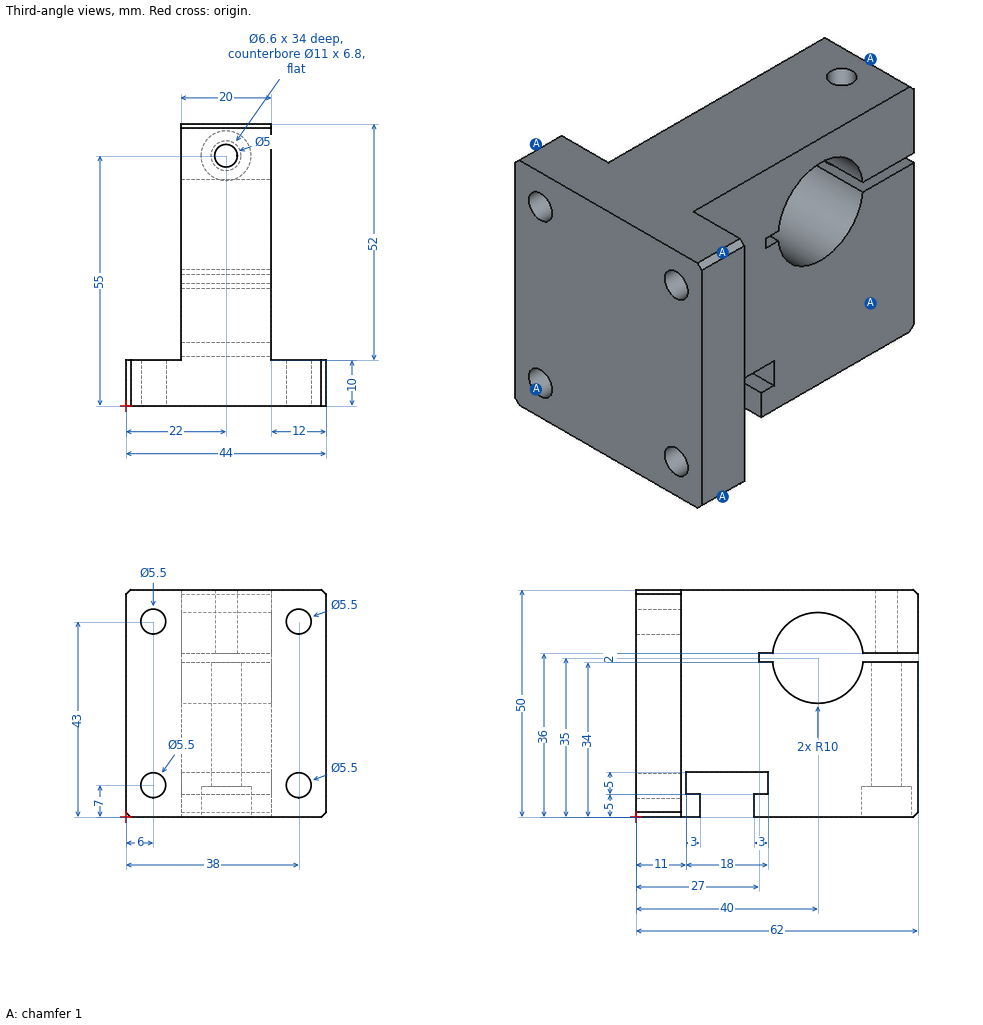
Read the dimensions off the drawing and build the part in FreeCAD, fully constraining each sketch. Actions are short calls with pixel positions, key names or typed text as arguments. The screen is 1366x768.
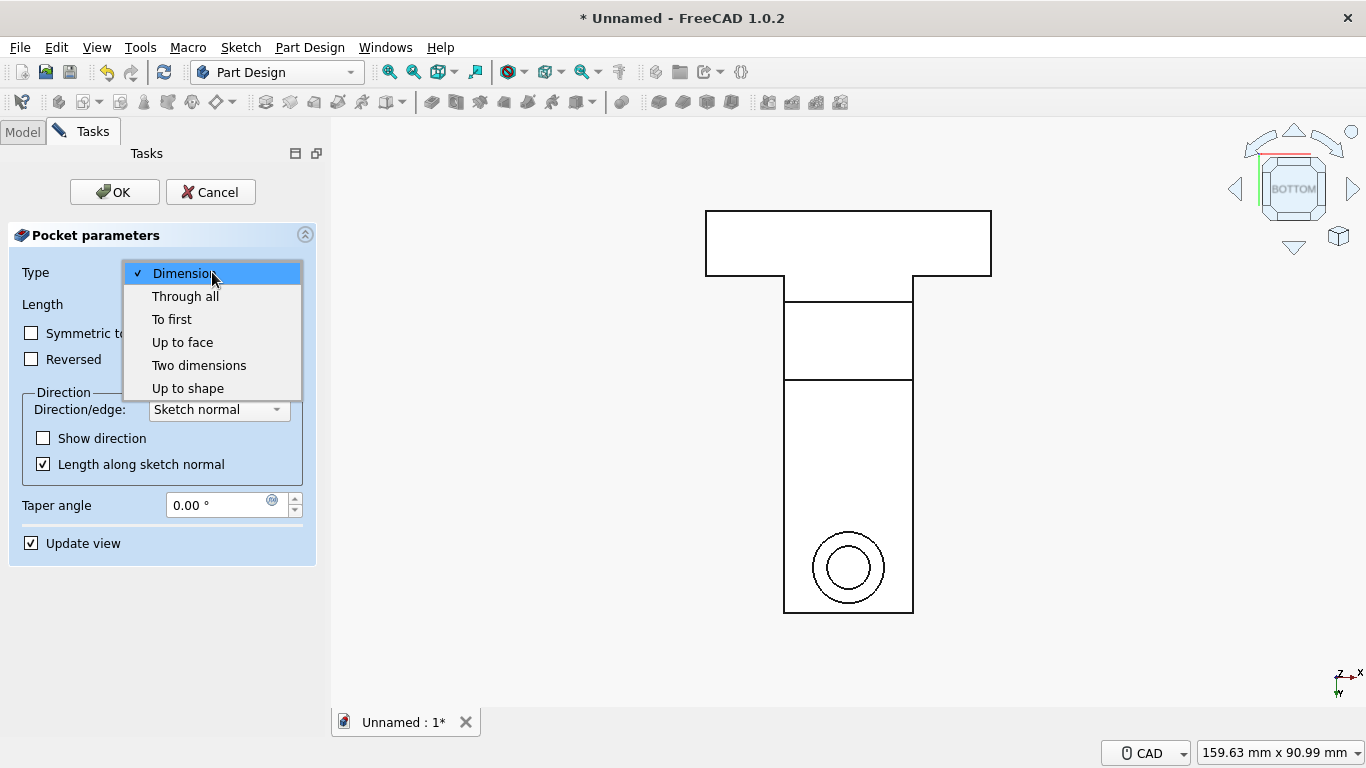
click(212, 296)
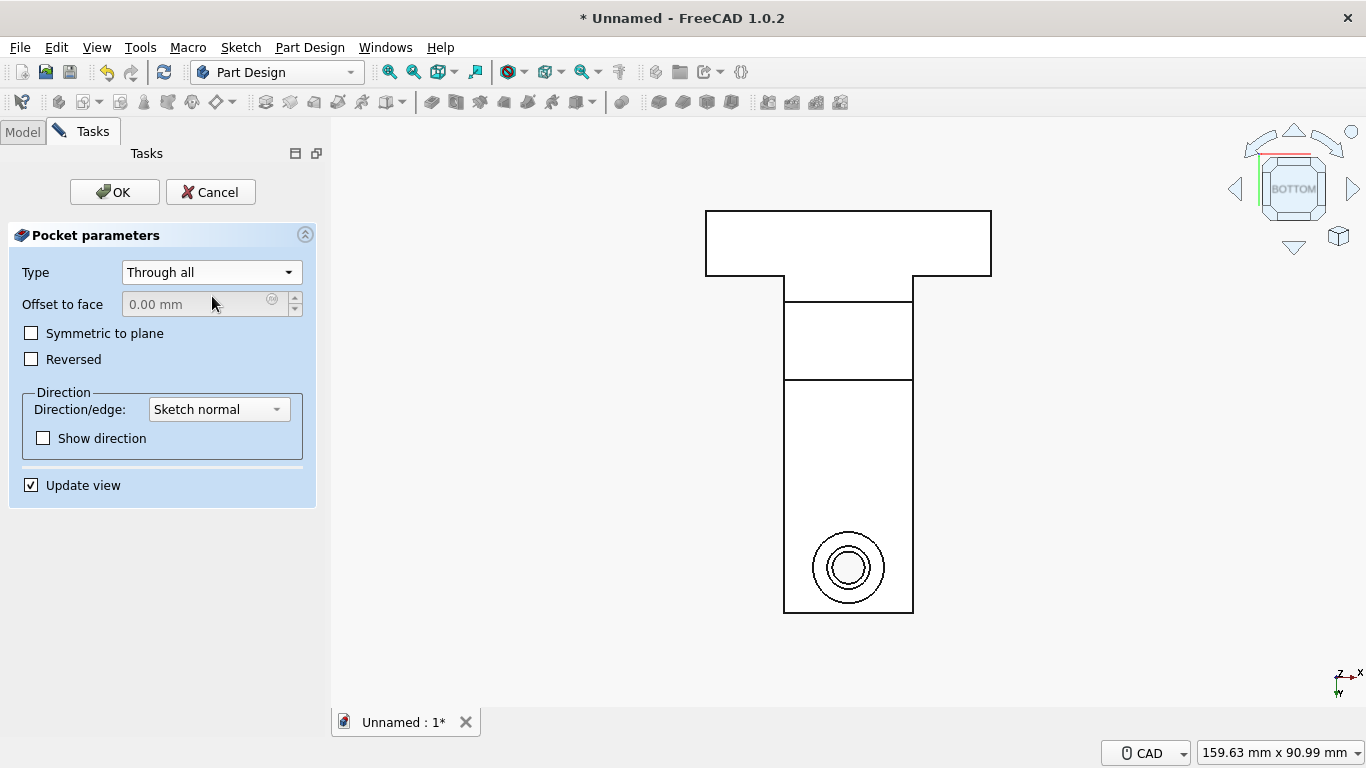
click(115, 192)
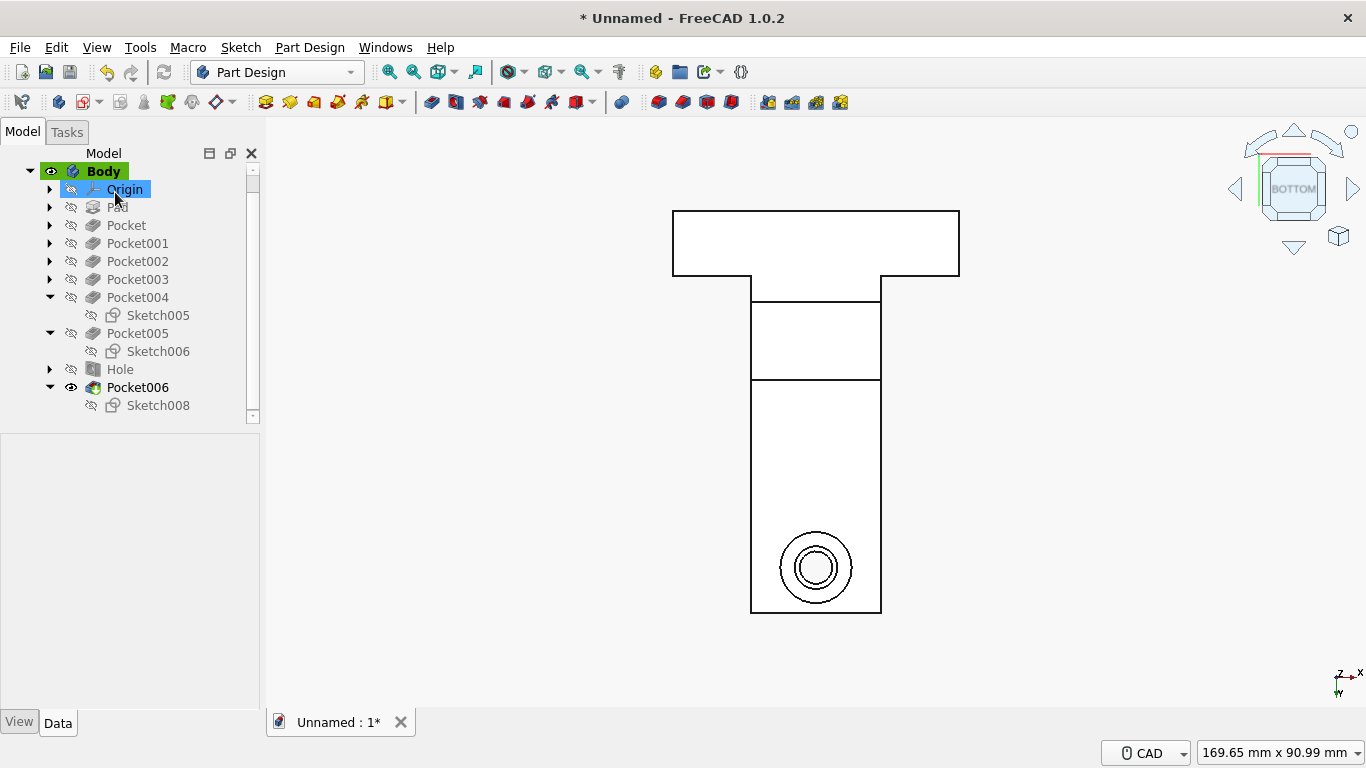
click(673, 242)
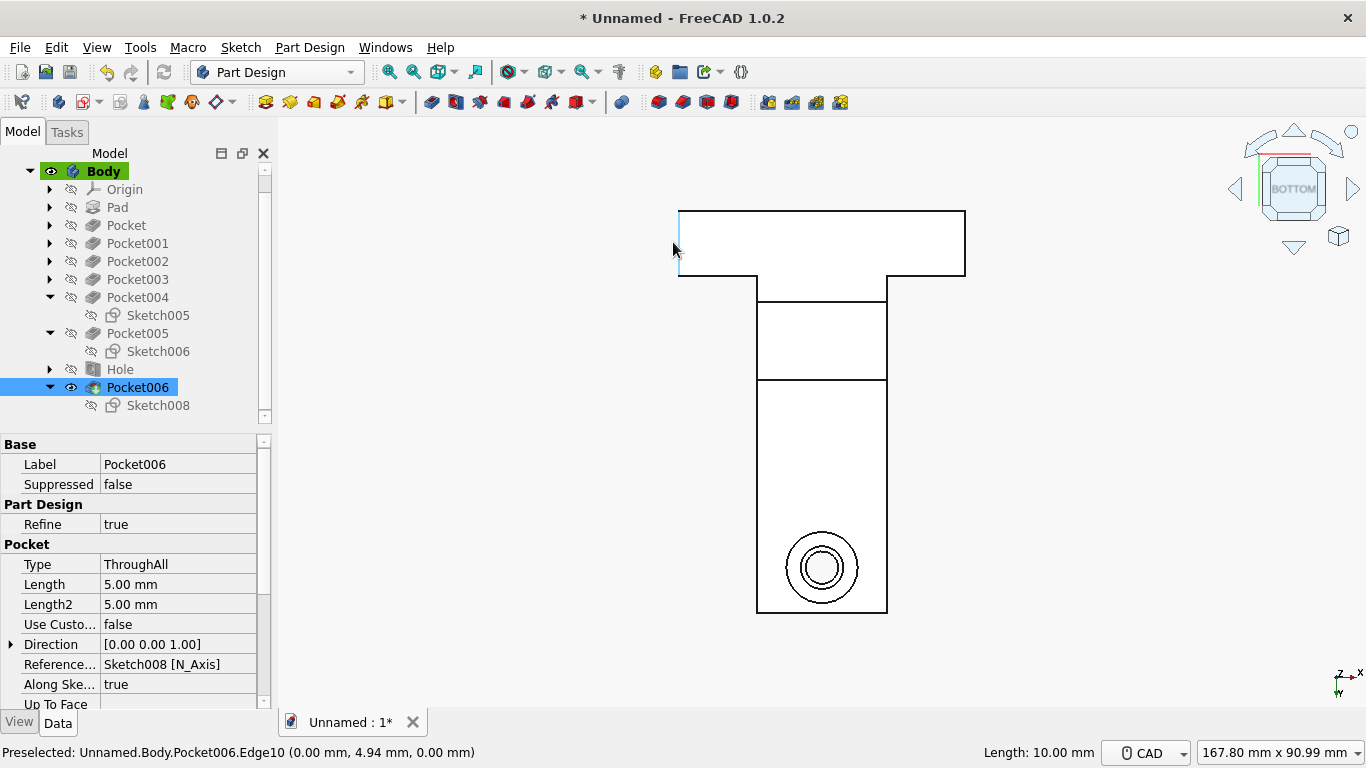
click(822, 612, ctrl)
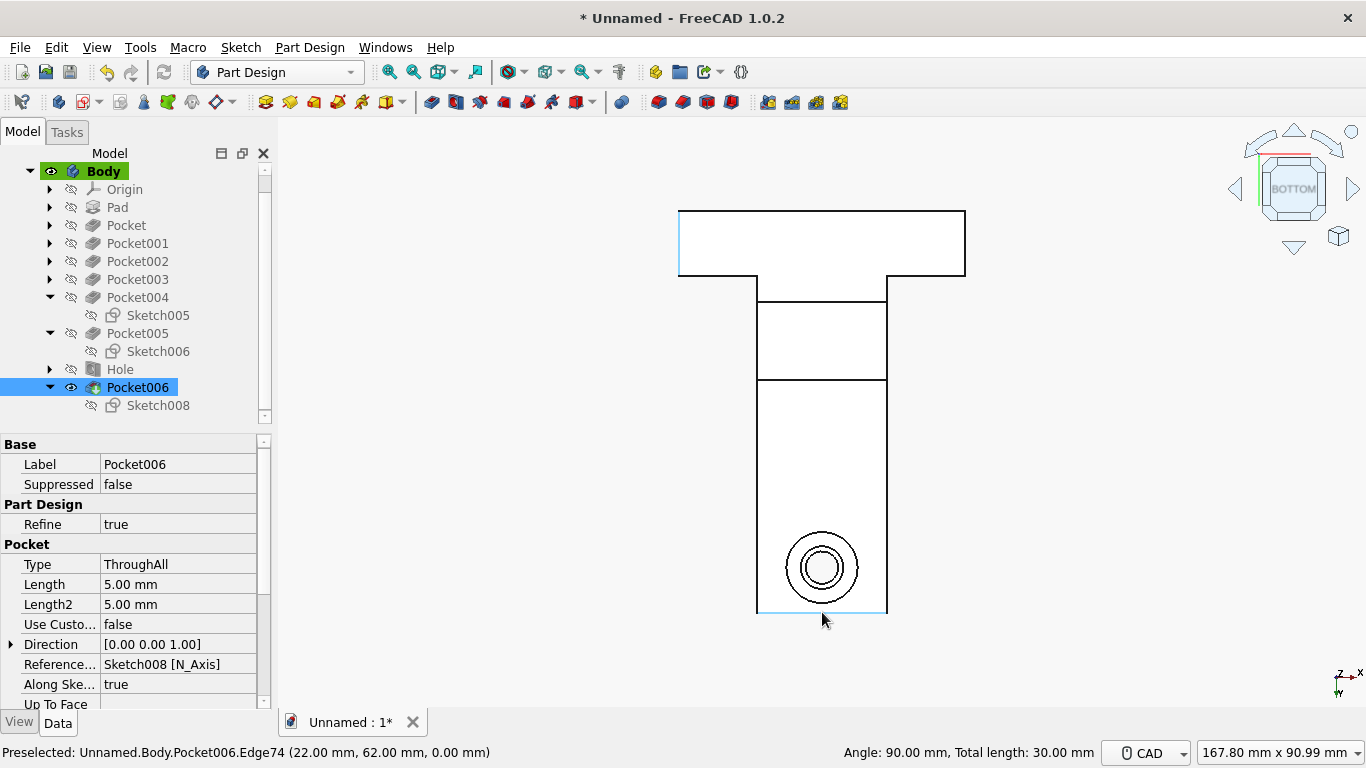
click(965, 242, ctrl)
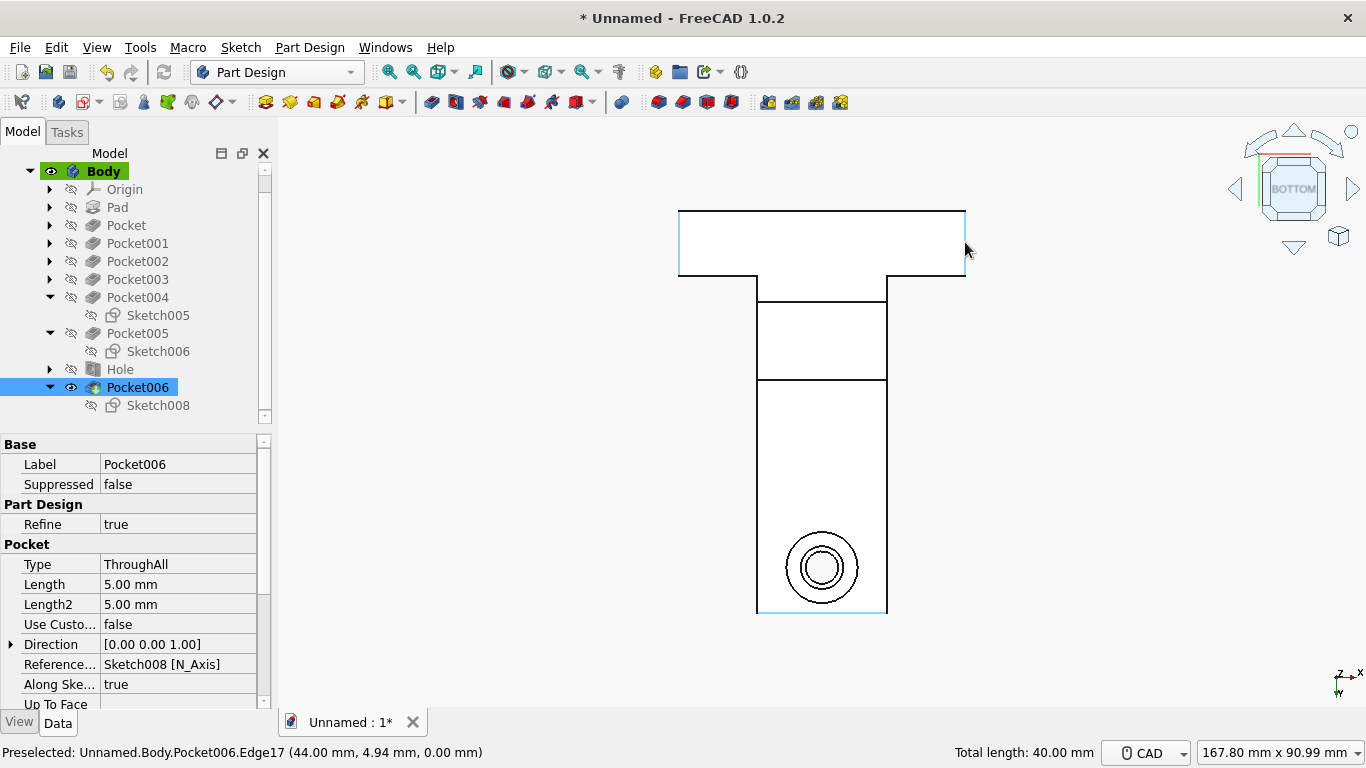
key(0)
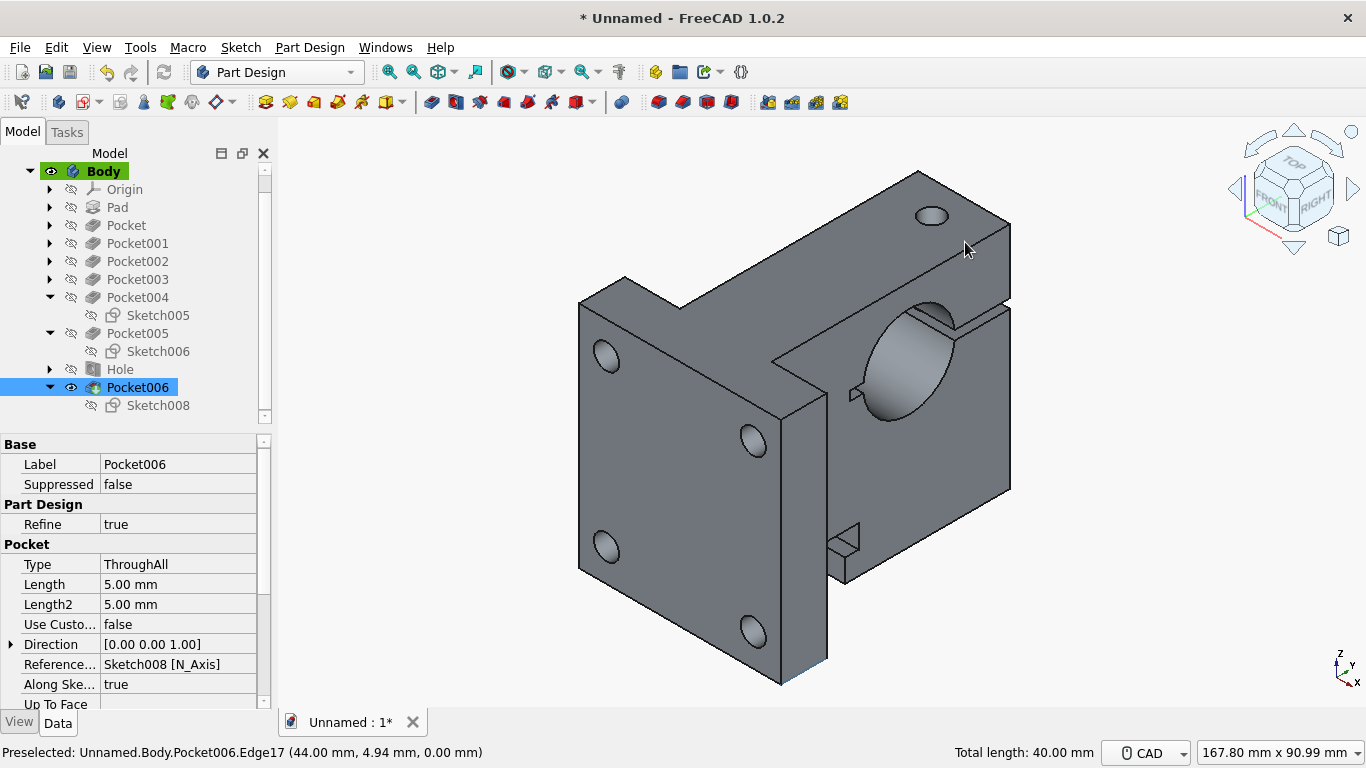
click(804, 406, ctrl)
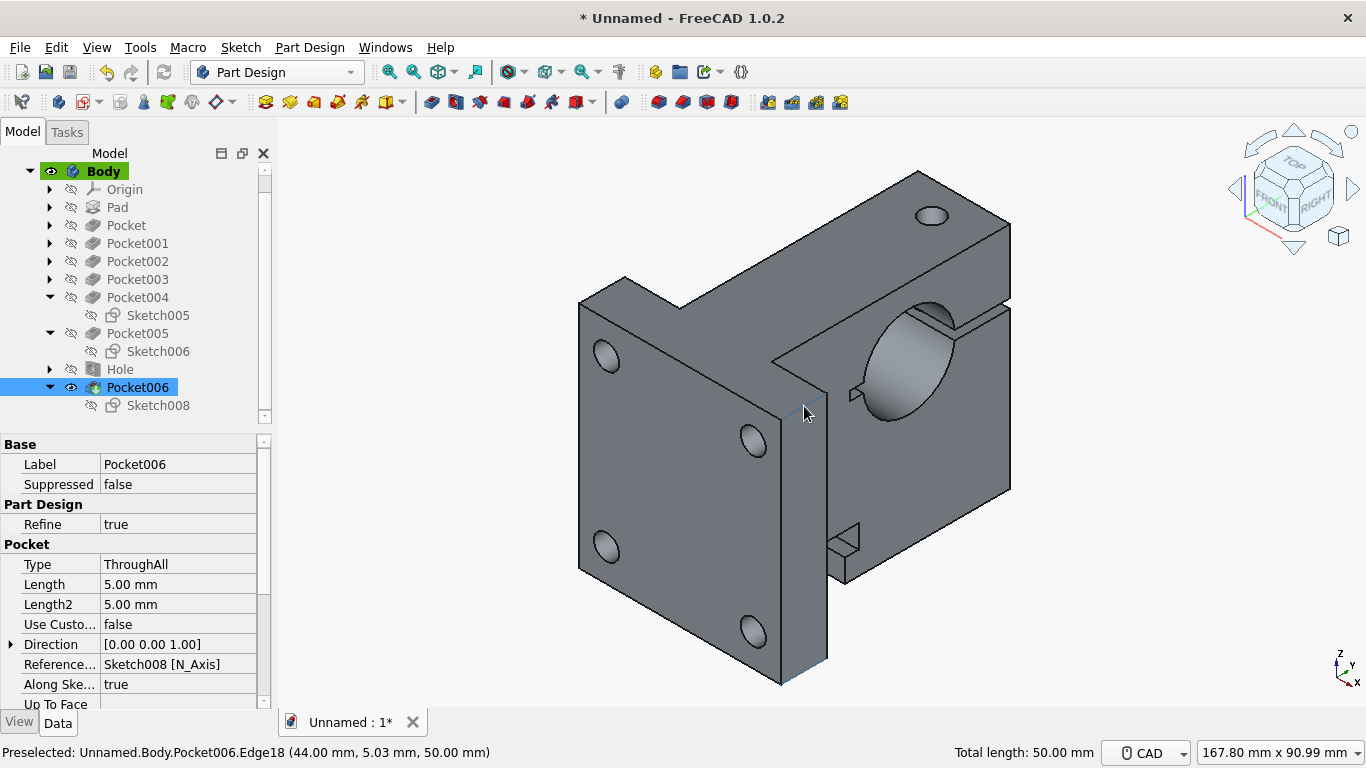
key(2)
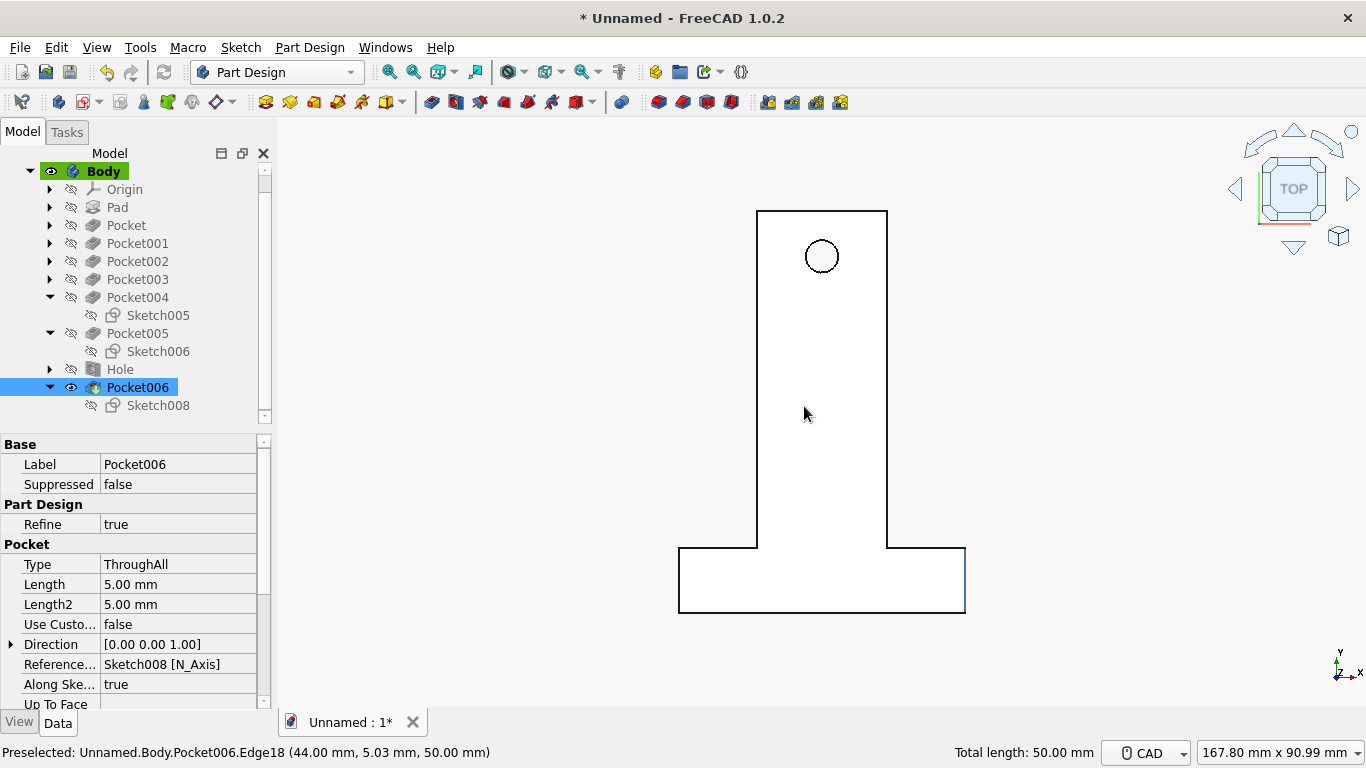
click(822, 210, ctrl)